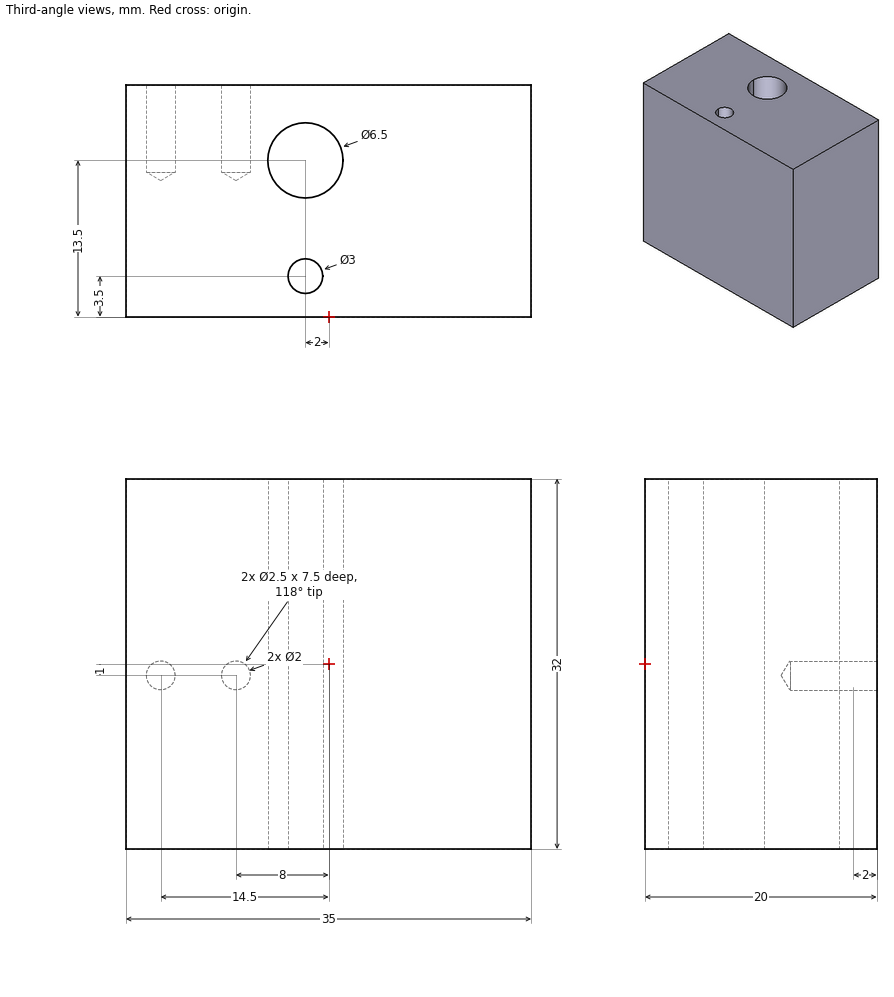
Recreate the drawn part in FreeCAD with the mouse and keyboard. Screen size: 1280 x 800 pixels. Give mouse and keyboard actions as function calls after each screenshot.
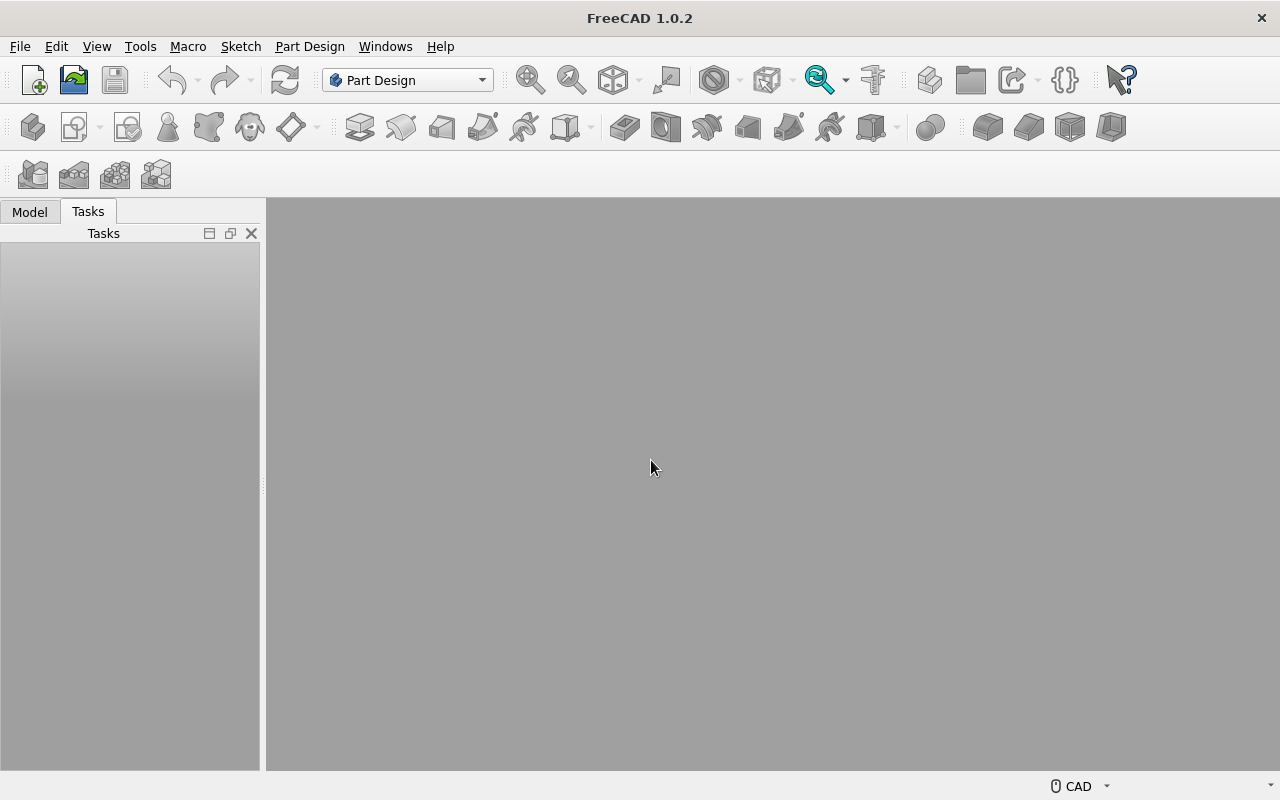
key(ctrl+n)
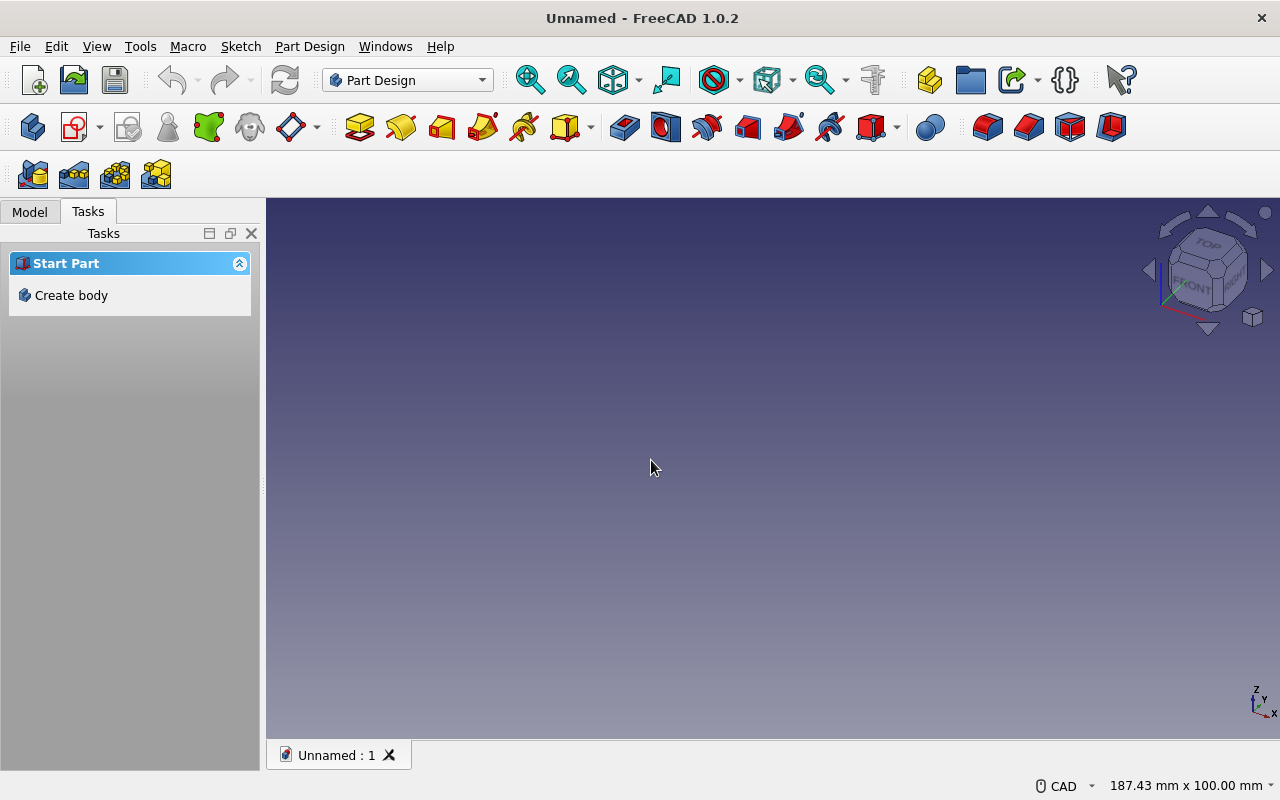
click(74, 128)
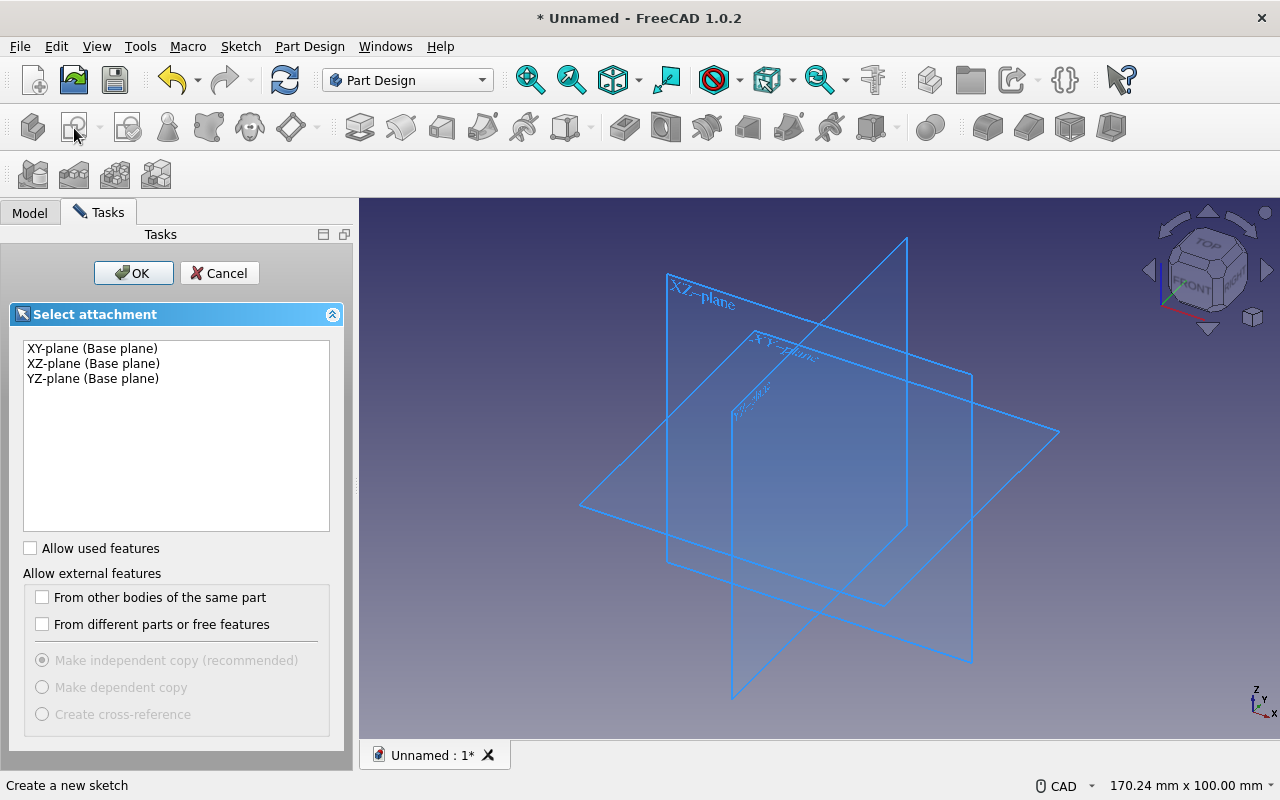
click(84, 364)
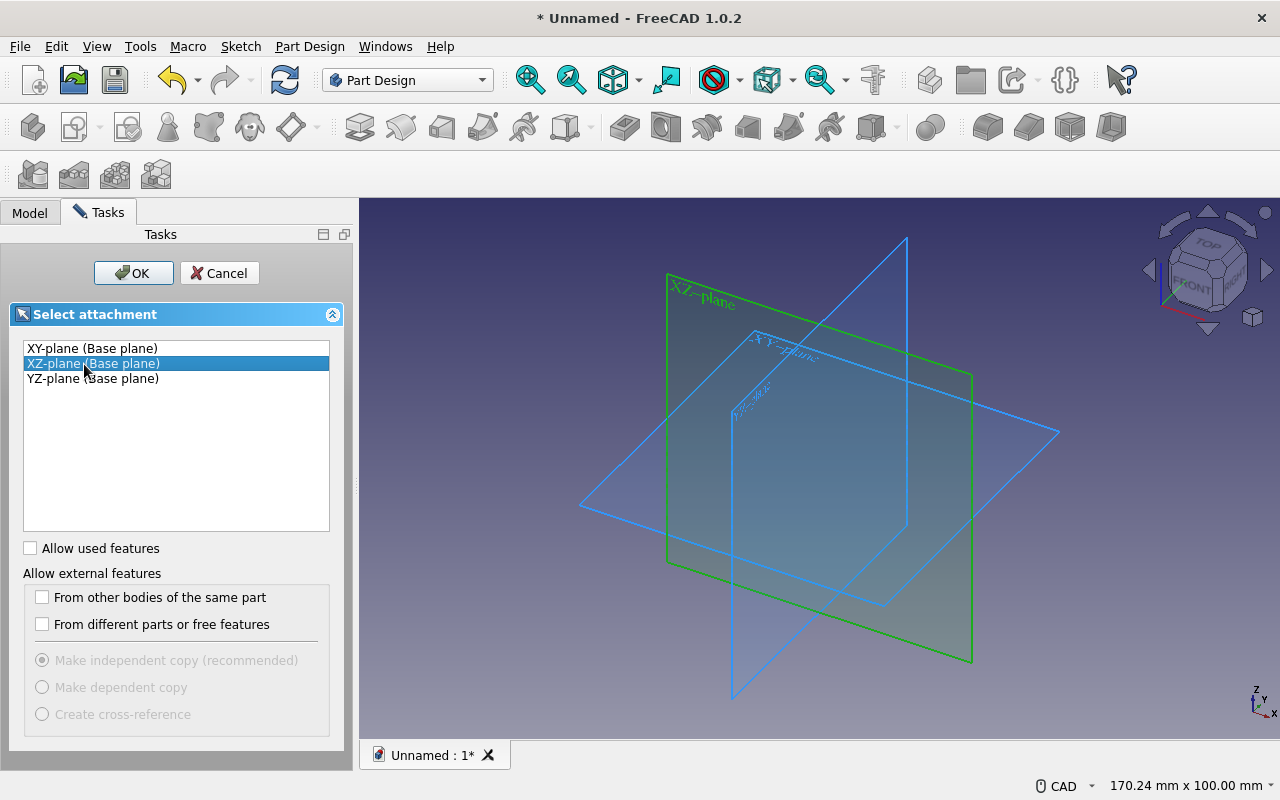
click(134, 273)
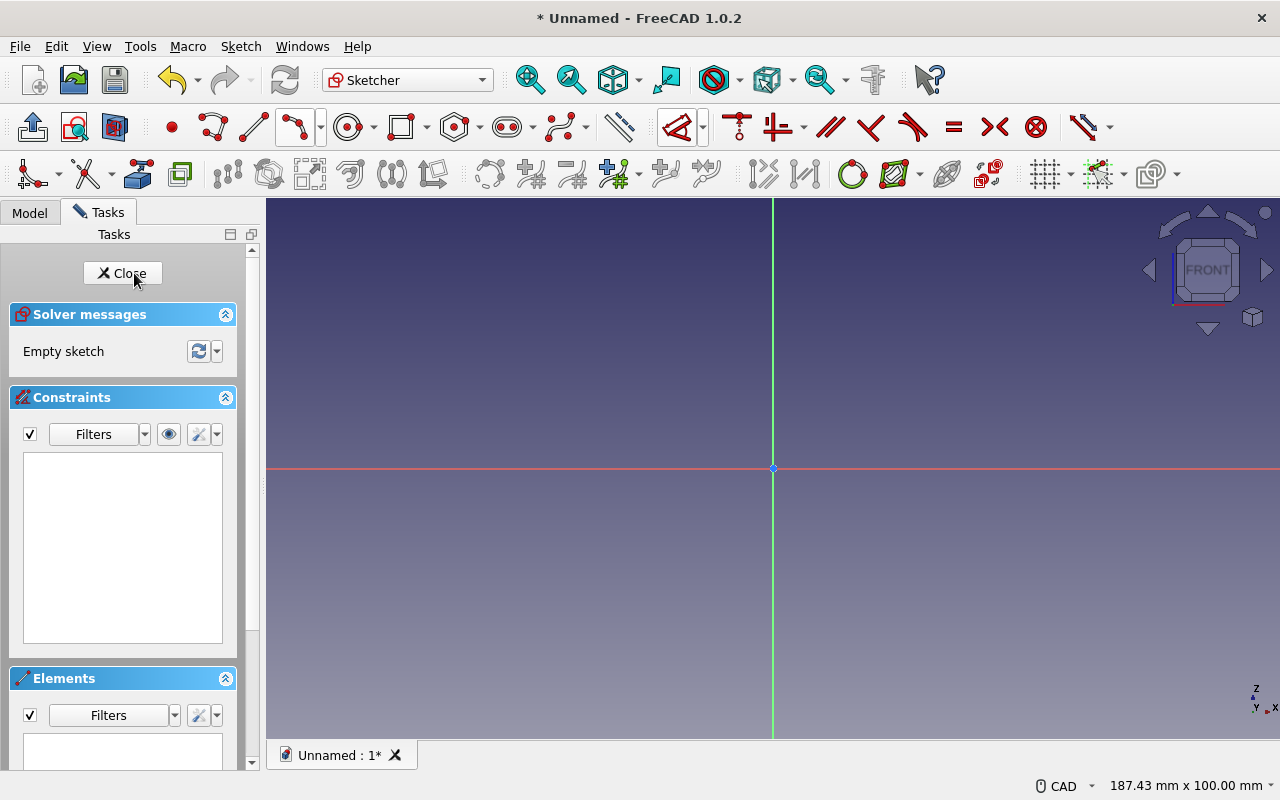
scroll(856, 468, up, 3)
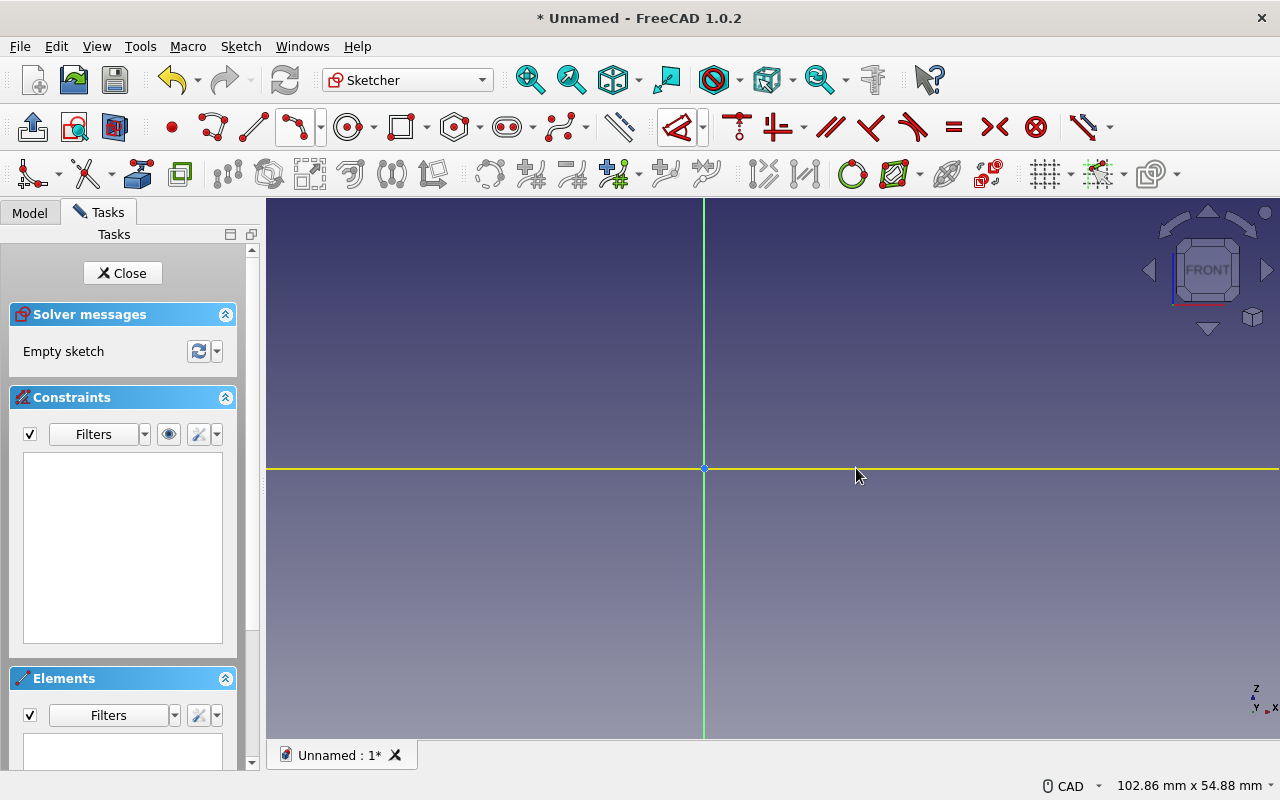
key(g)
key(v)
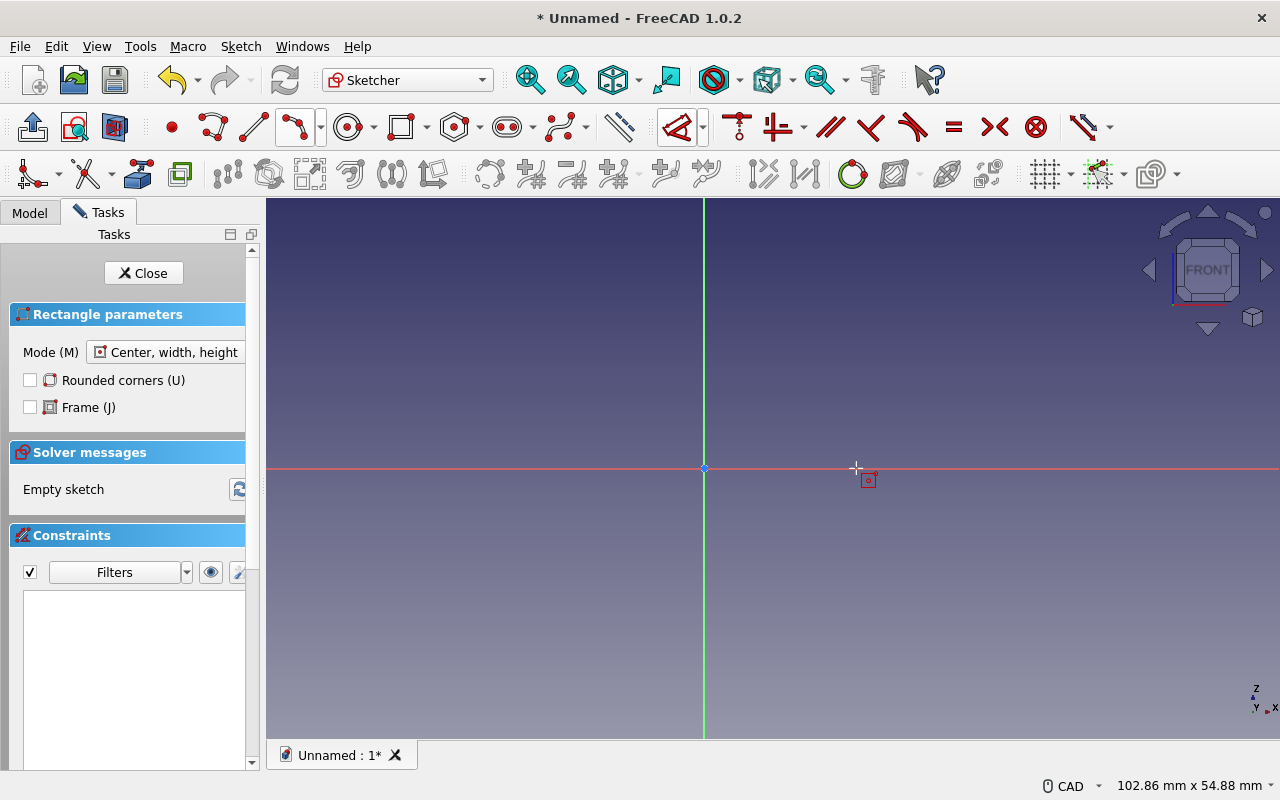
click(704, 468)
click(877, 311)
key(Escape)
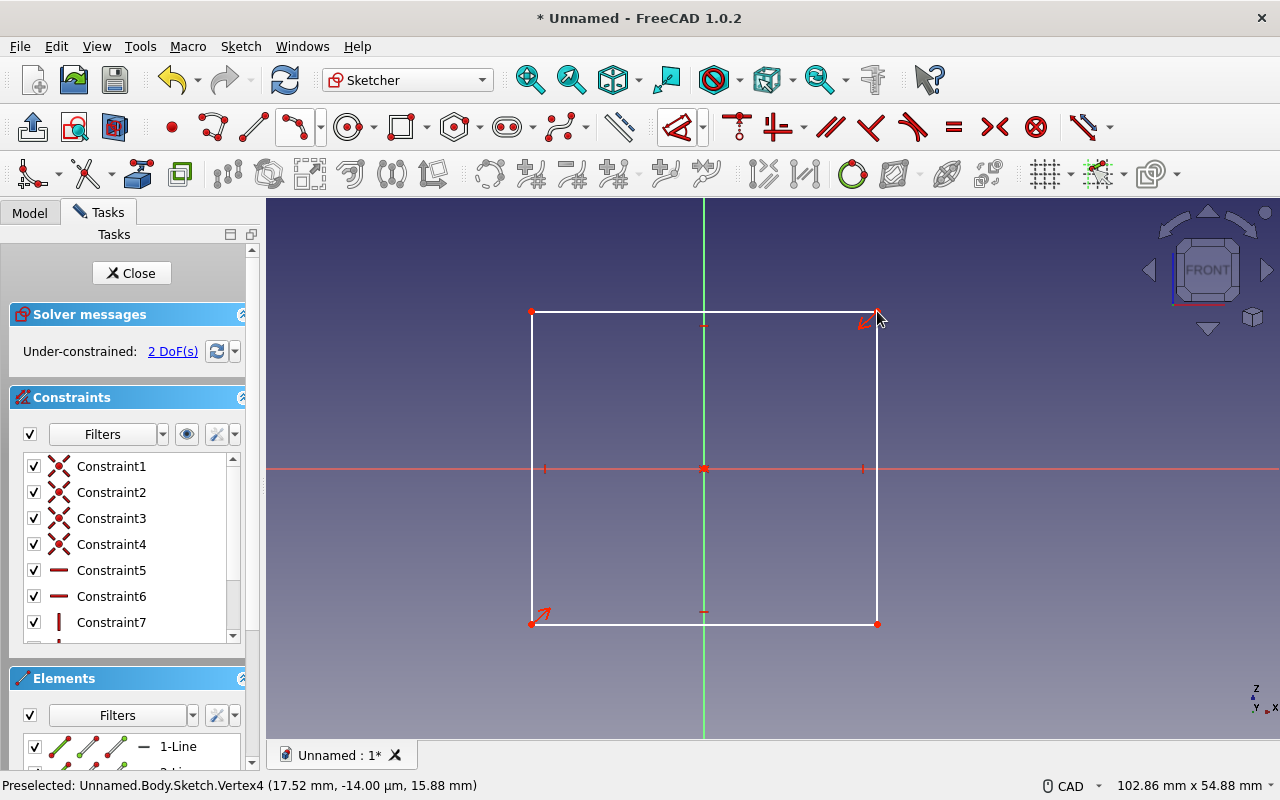
click(635, 625)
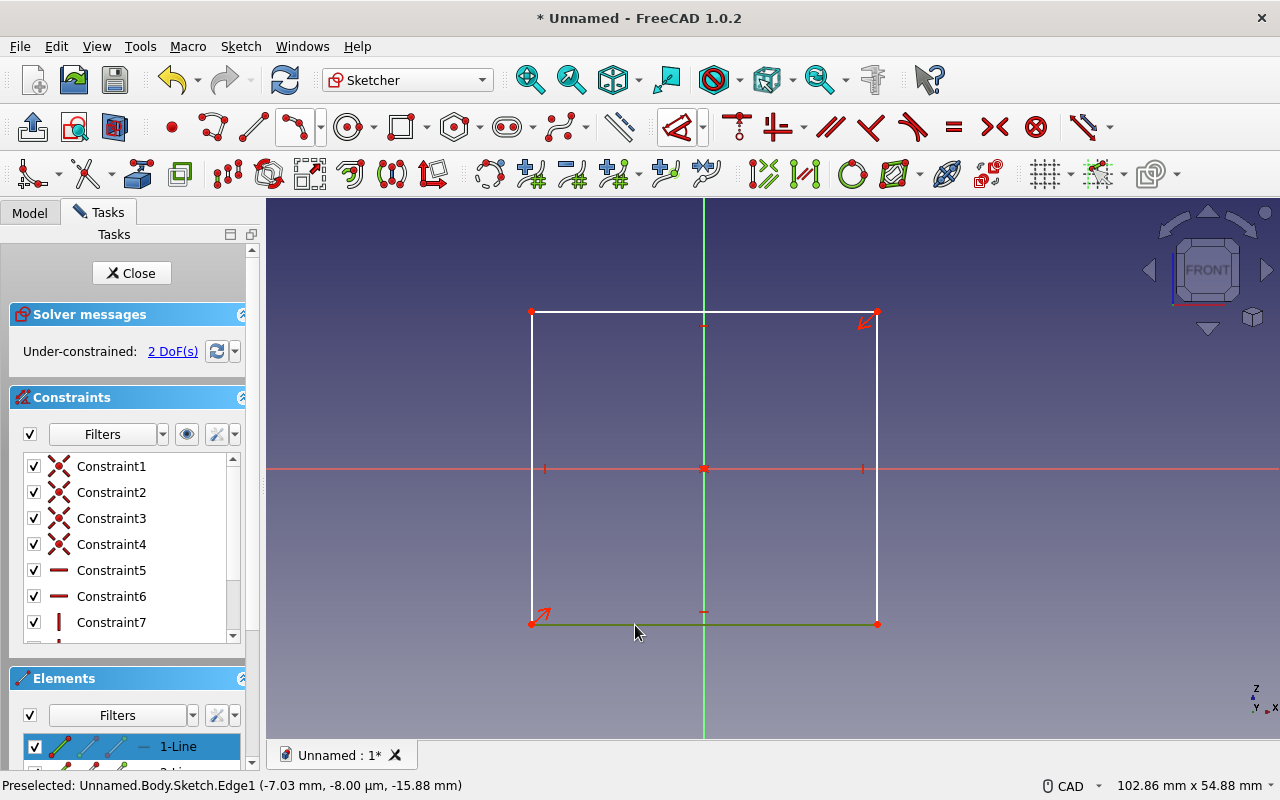
key(l)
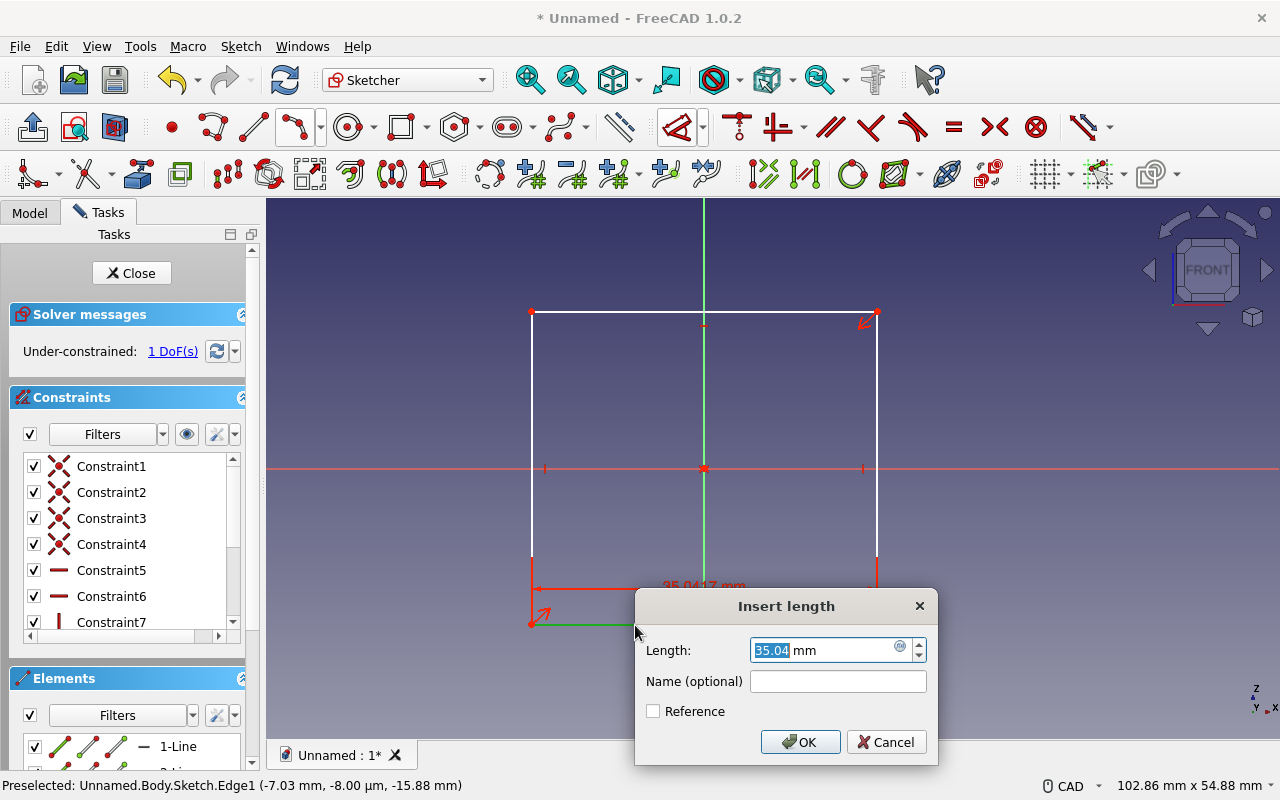
text(35)
key(Return)